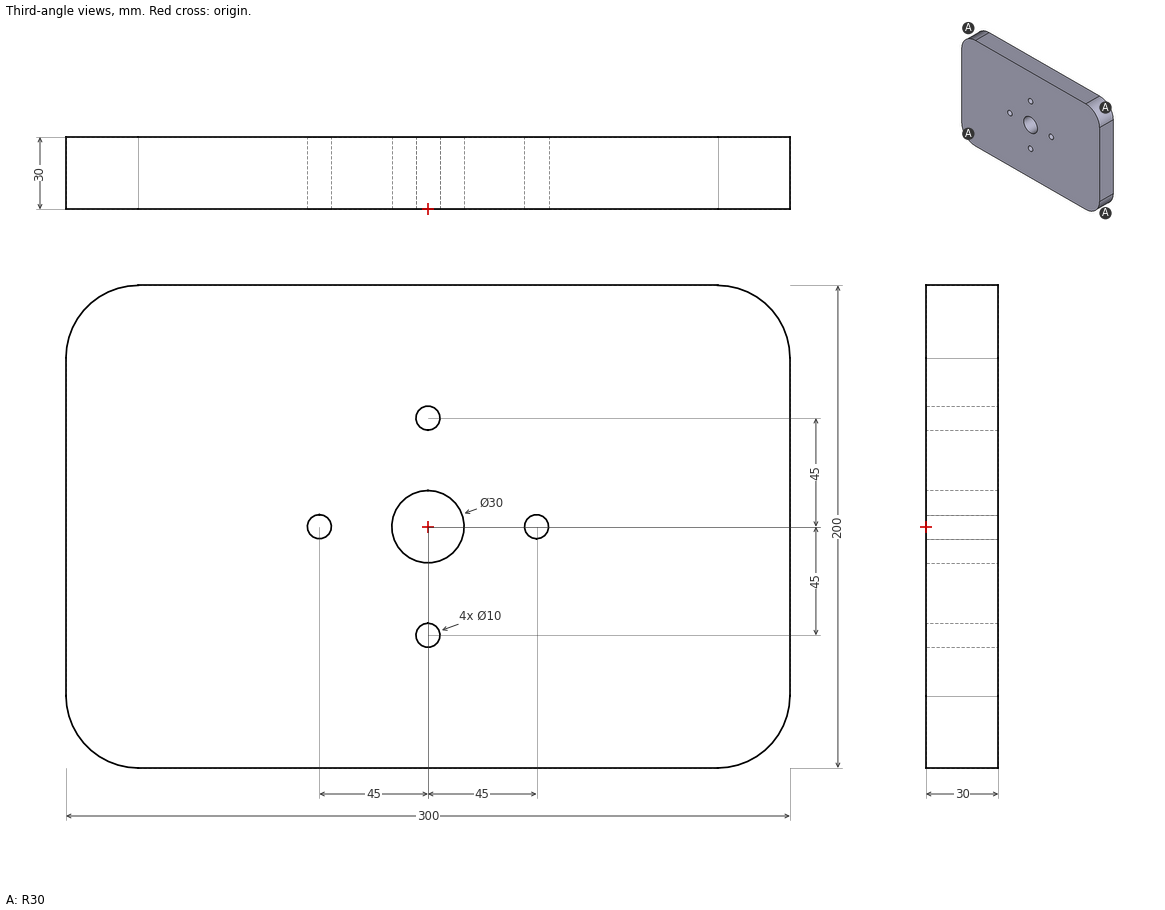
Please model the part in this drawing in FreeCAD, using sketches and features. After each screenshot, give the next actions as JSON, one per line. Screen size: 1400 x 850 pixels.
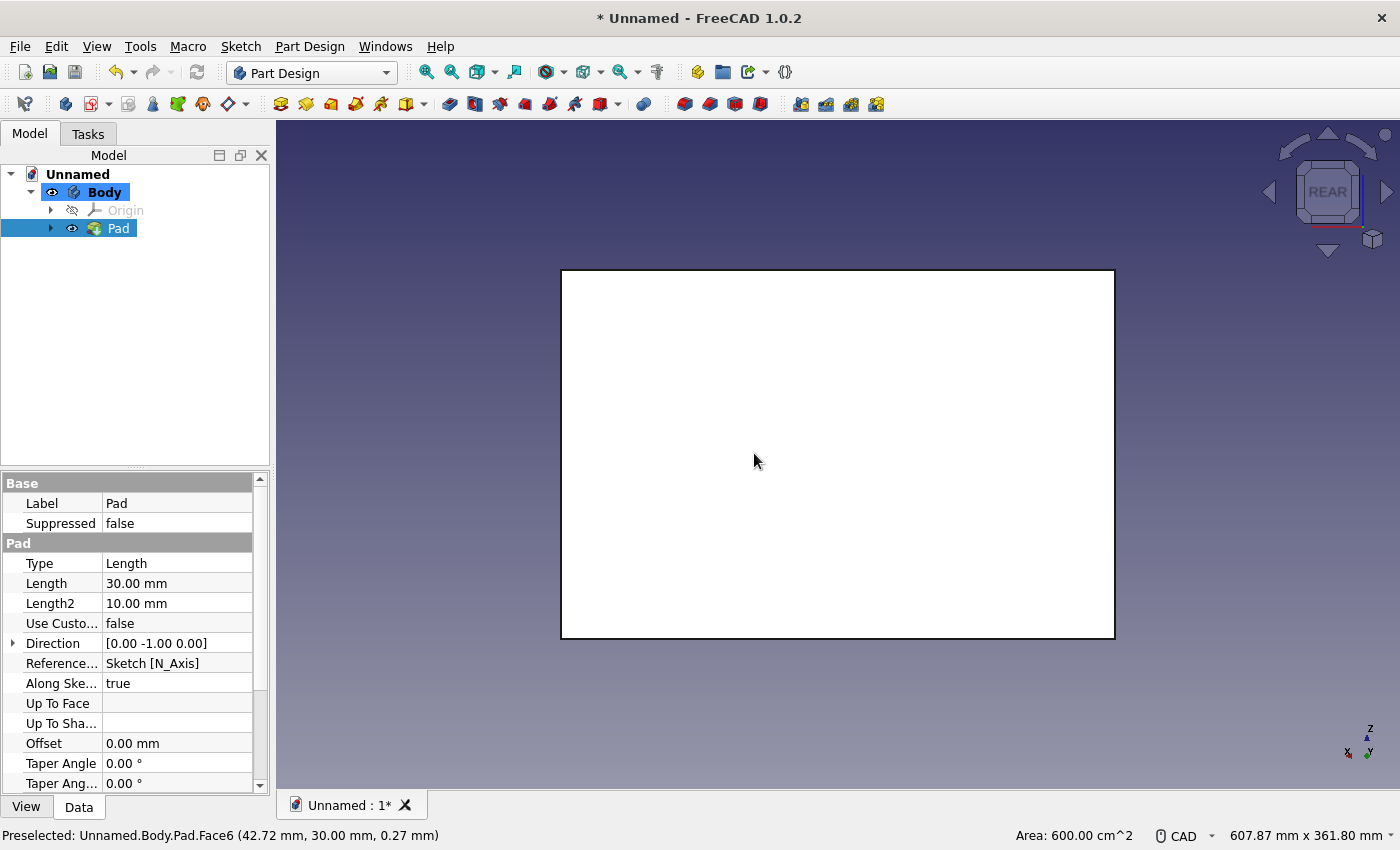
{"action": "left_click", "coordinate": [90, 104]}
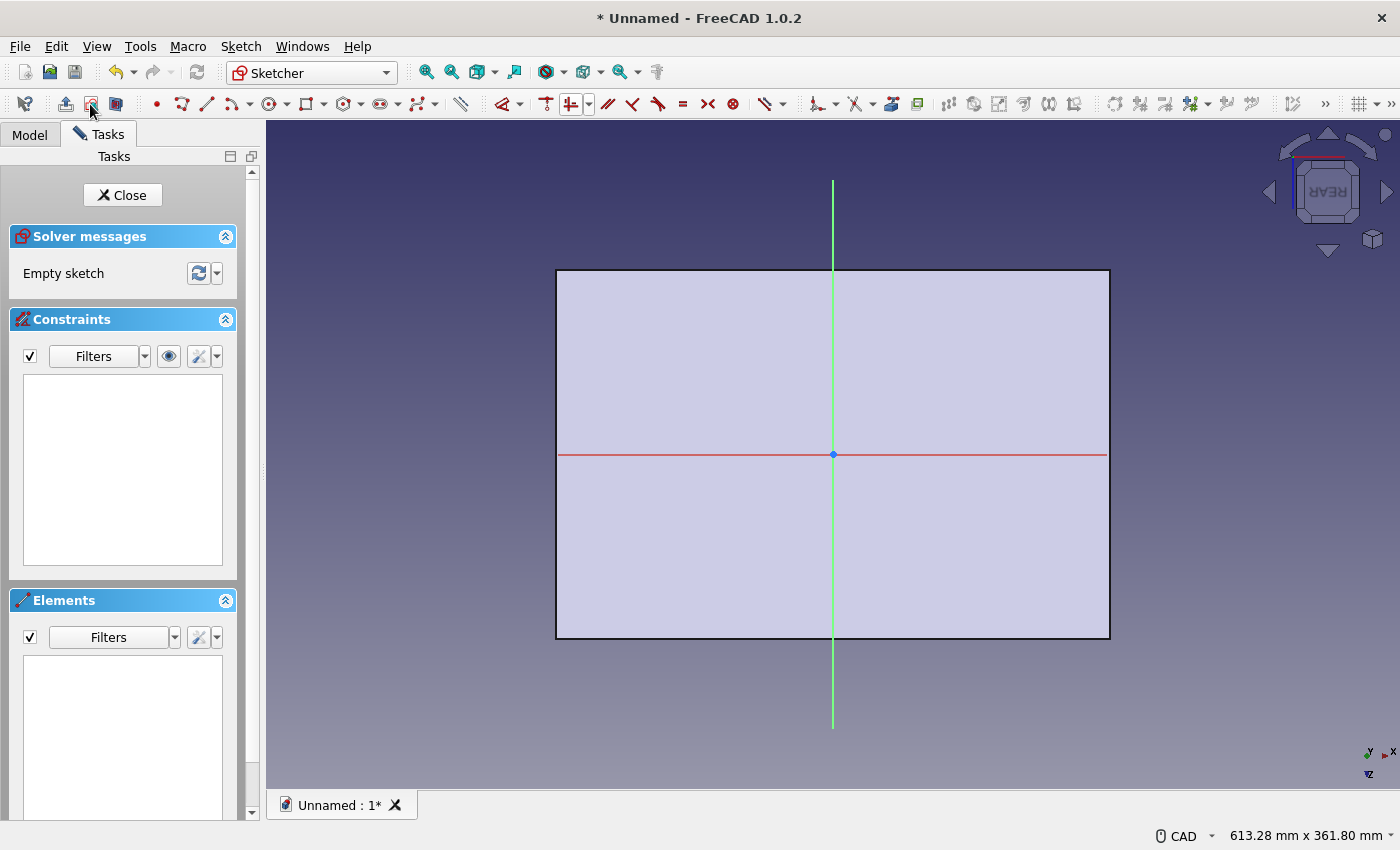
{"action": "scroll", "coordinate": [889, 455], "scroll_direction": "up", "scroll_amount": 4}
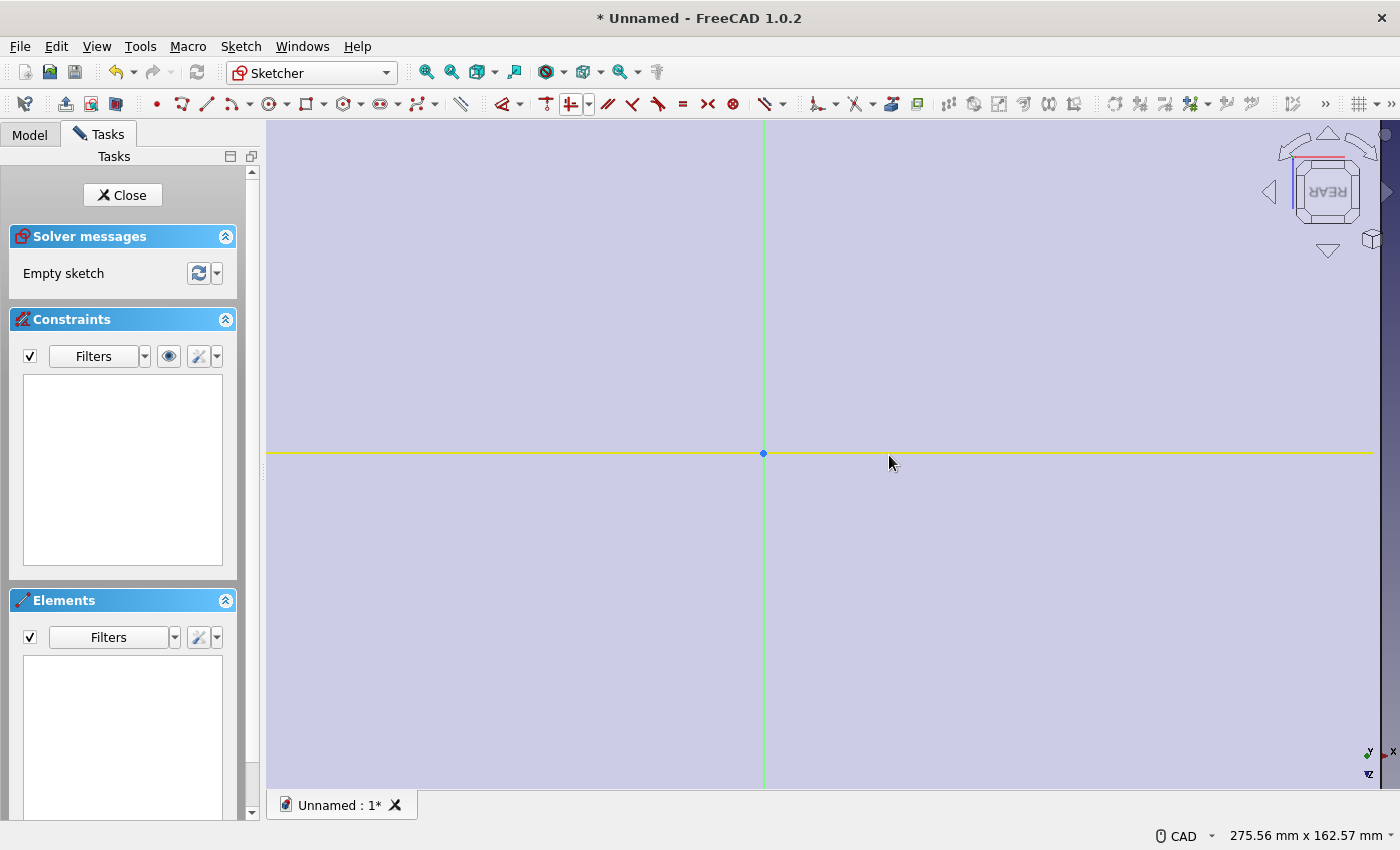
{"action": "key", "text": "g c"}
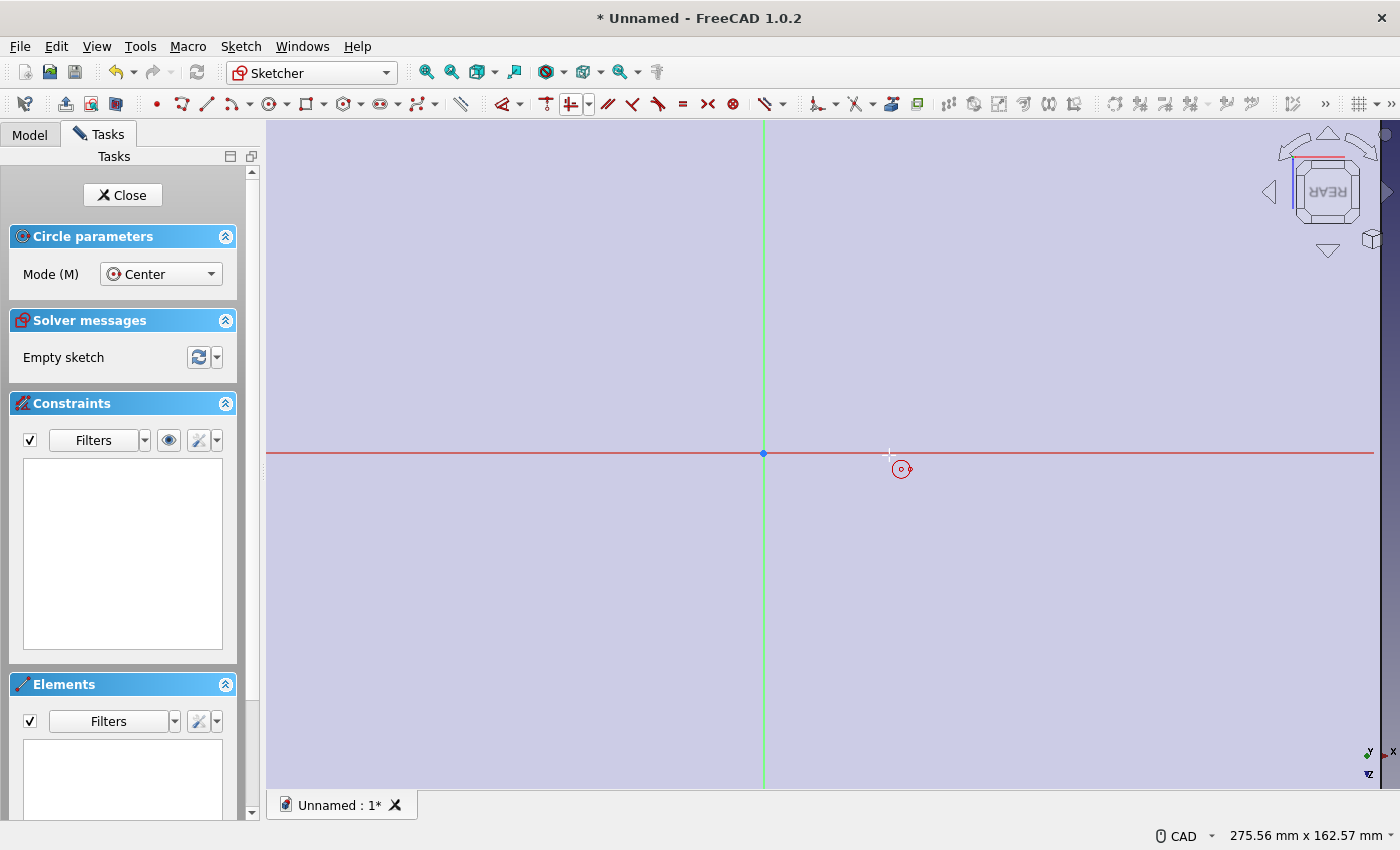
{"action": "left_click", "coordinate": [764, 453]}
{"action": "mouse_move", "coordinate": [807, 410]}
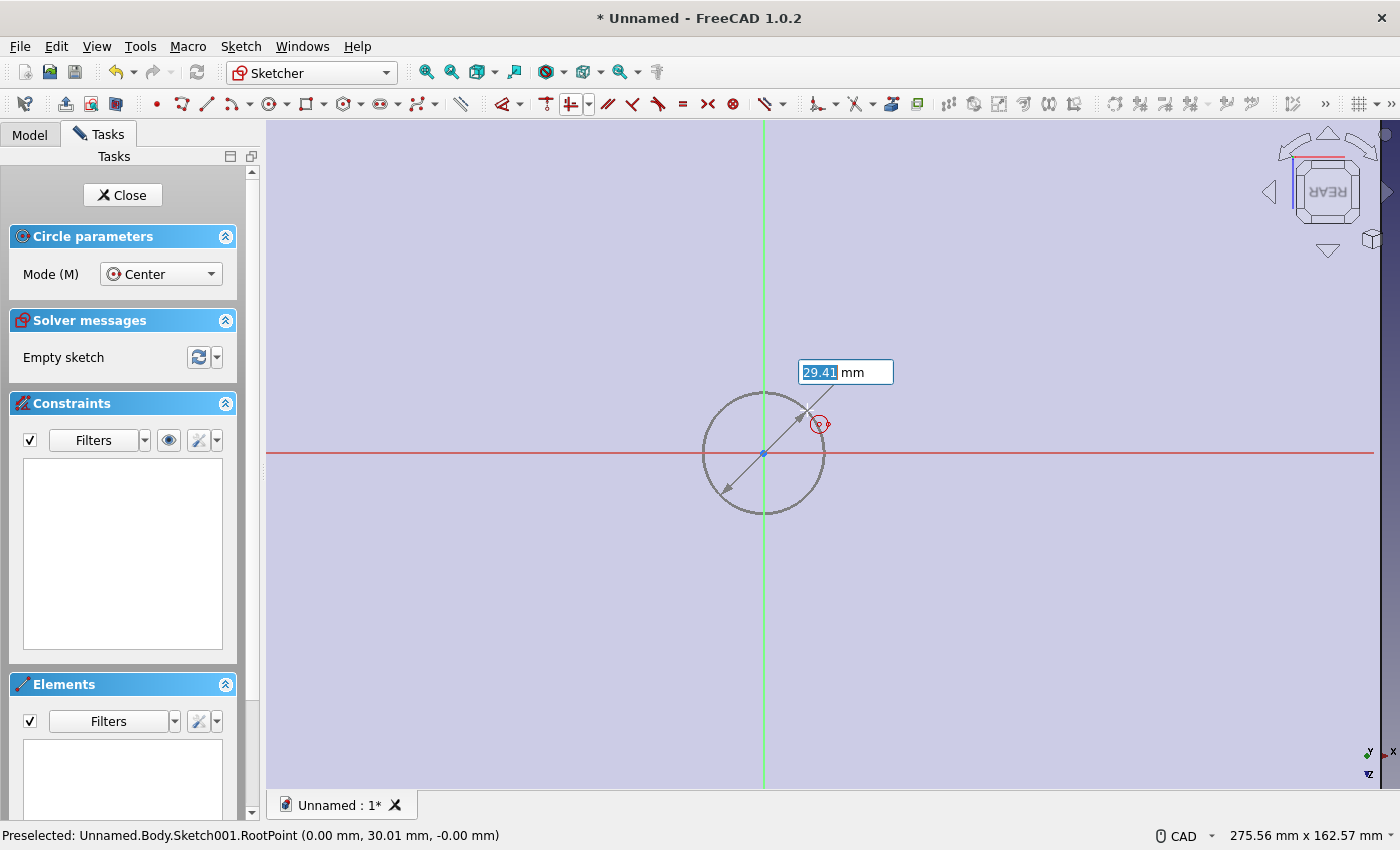
{"action": "type", "text": "30"}
{"action": "key", "text": "Return"}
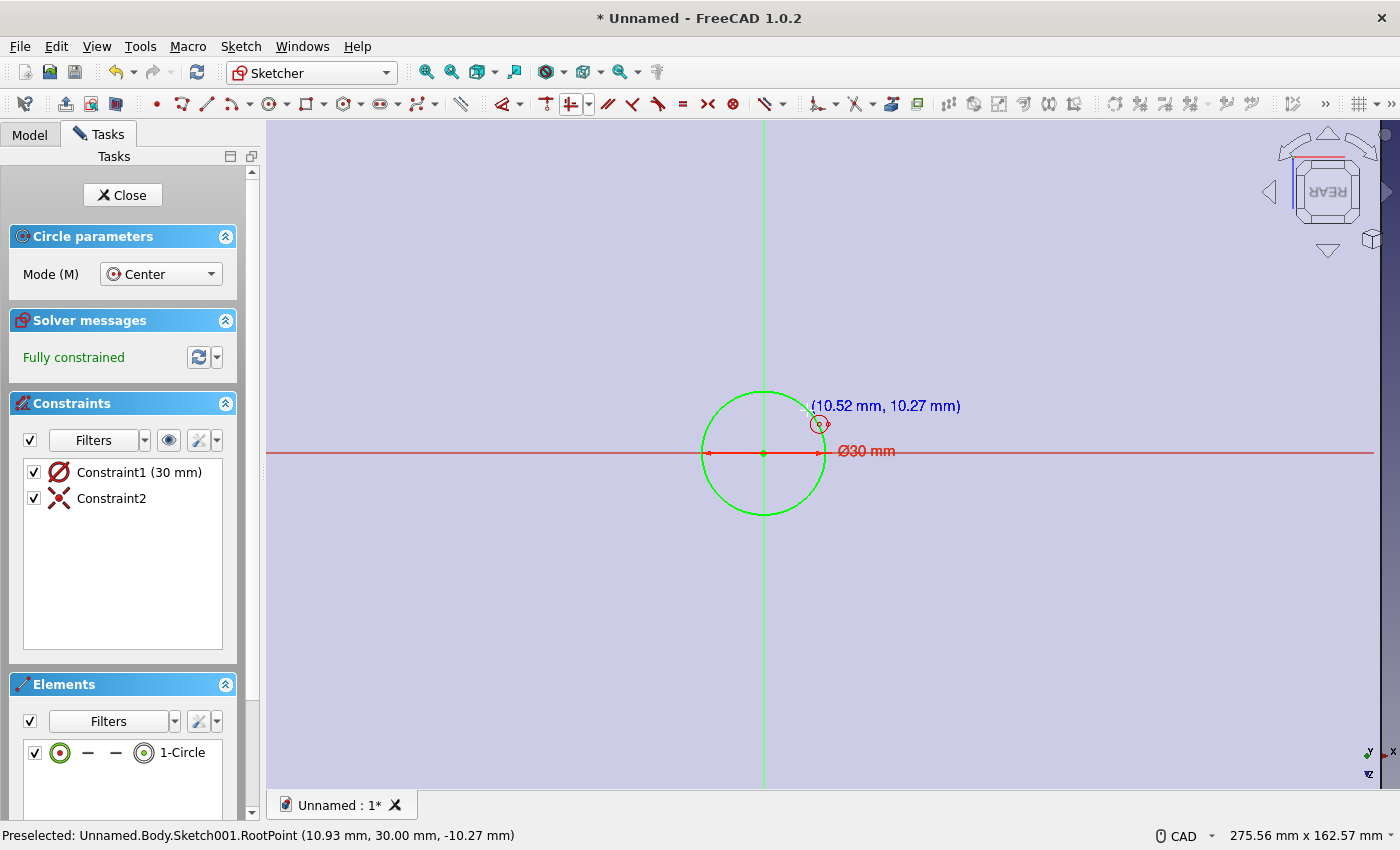
{"action": "left_click", "coordinate": [764, 268]}
{"action": "mouse_move", "coordinate": [778, 254]}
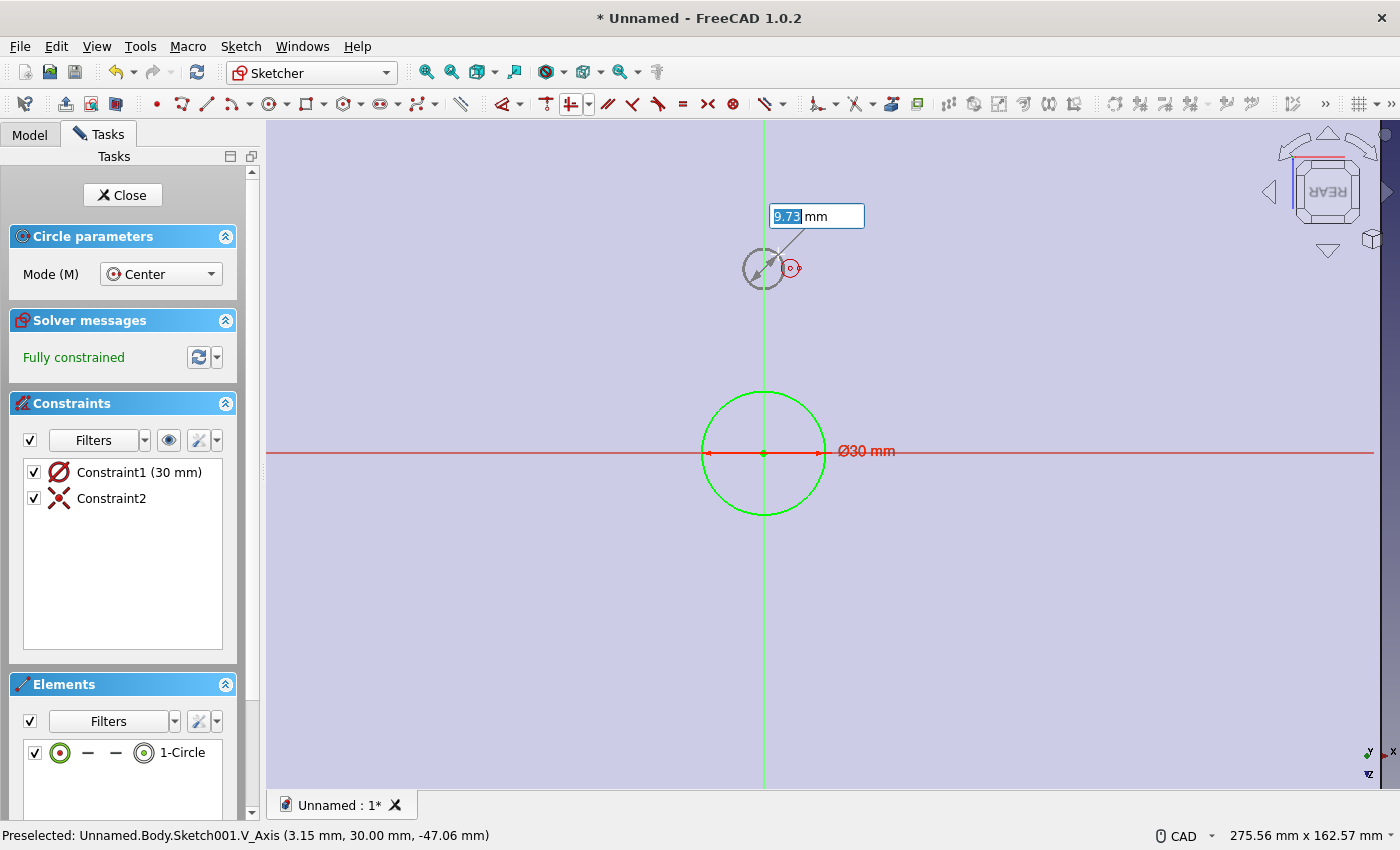
{"action": "type", "text": "10"}
{"action": "key", "text": "Return"}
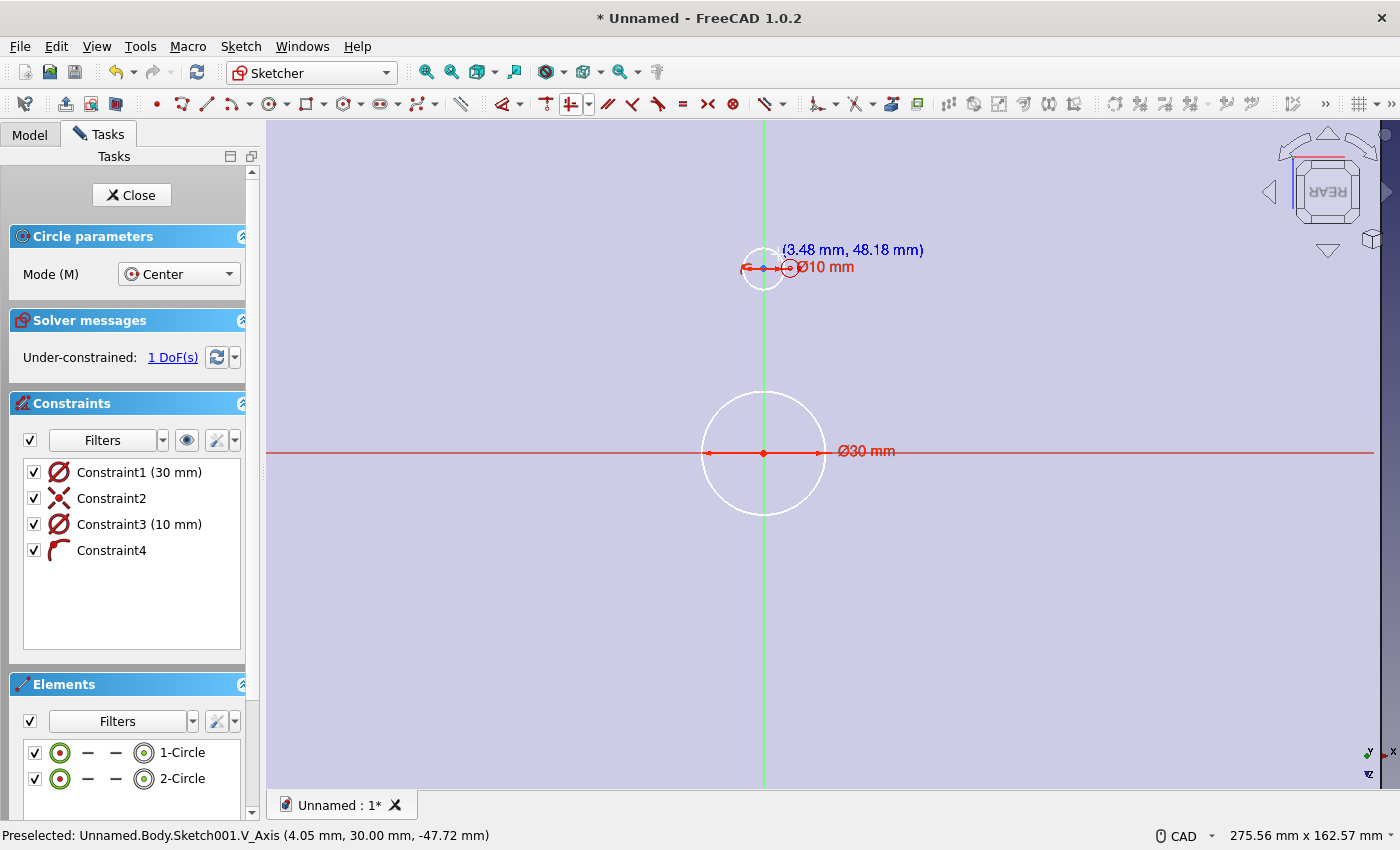
{"action": "left_click", "coordinate": [579, 453]}
{"action": "mouse_move", "coordinate": [593, 439]}